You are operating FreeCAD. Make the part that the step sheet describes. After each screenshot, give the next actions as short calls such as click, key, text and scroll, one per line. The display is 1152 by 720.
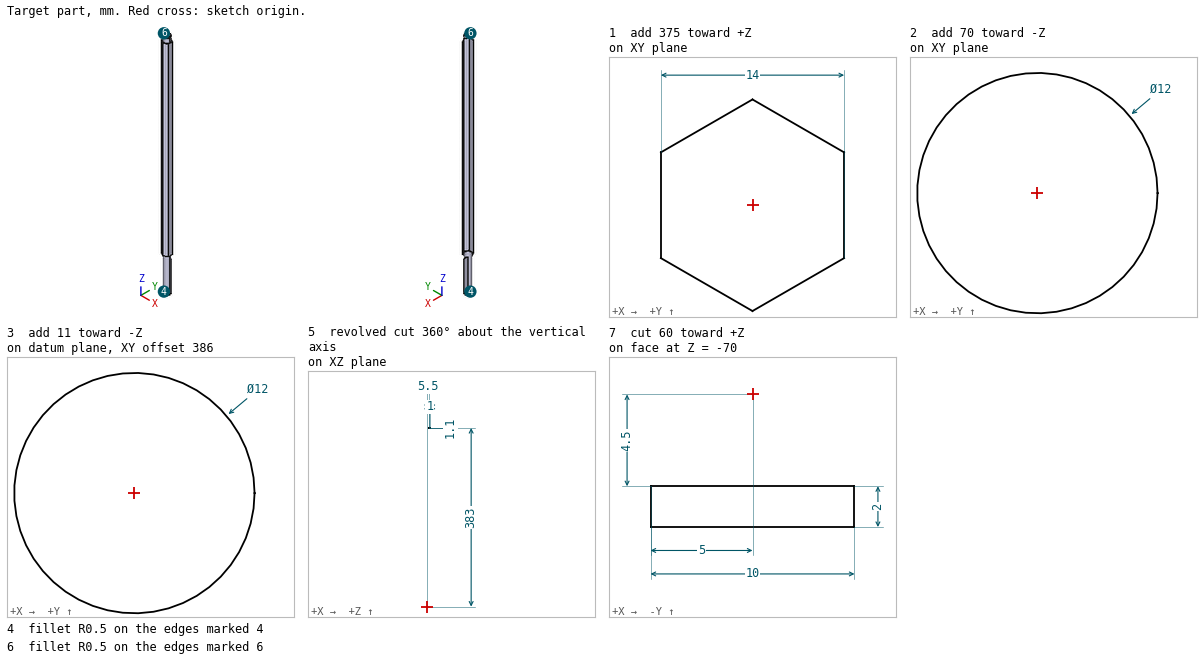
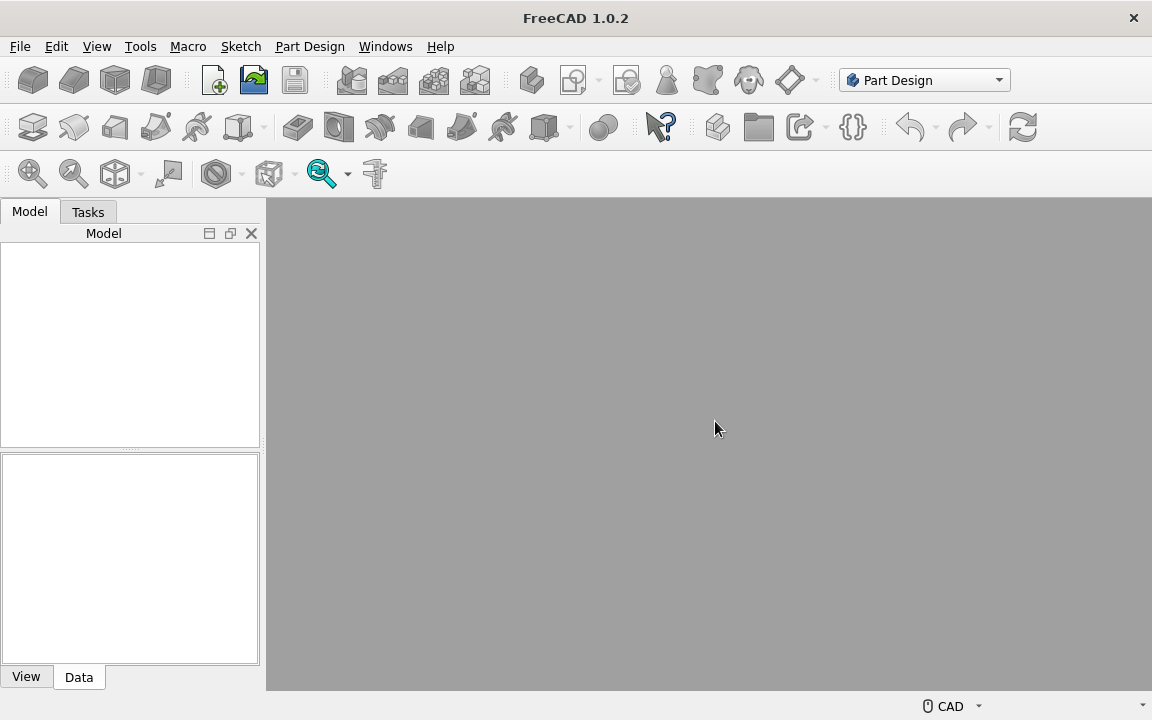
click(213, 80)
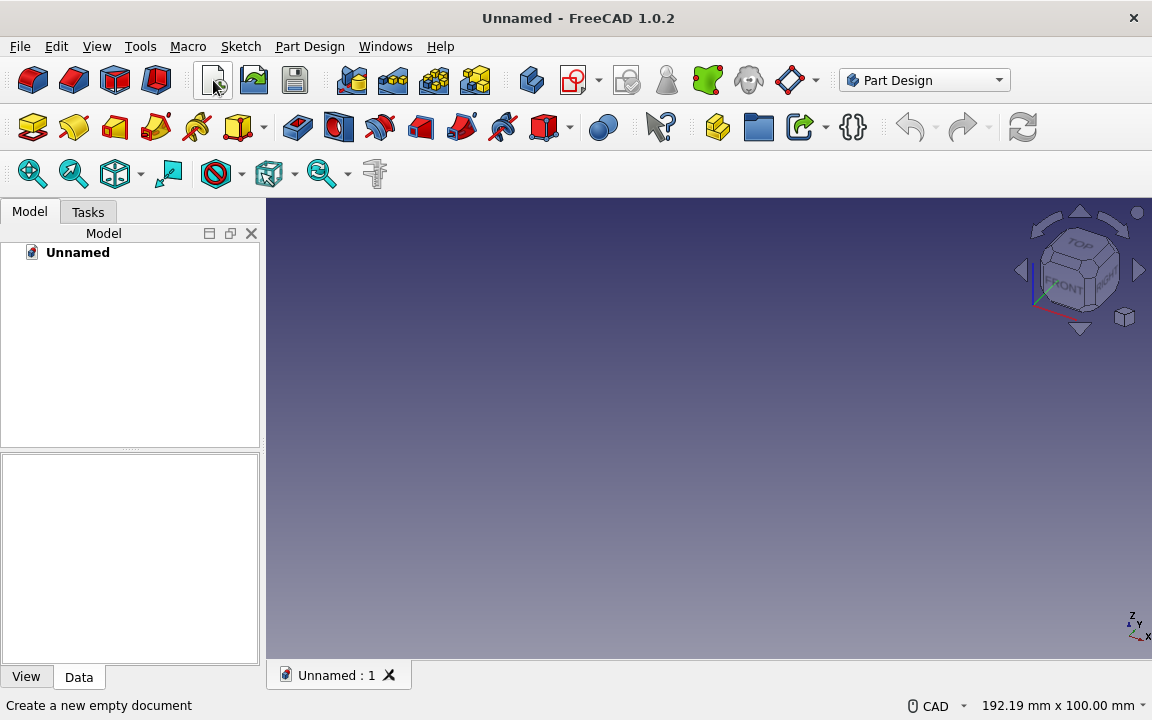
click(572, 80)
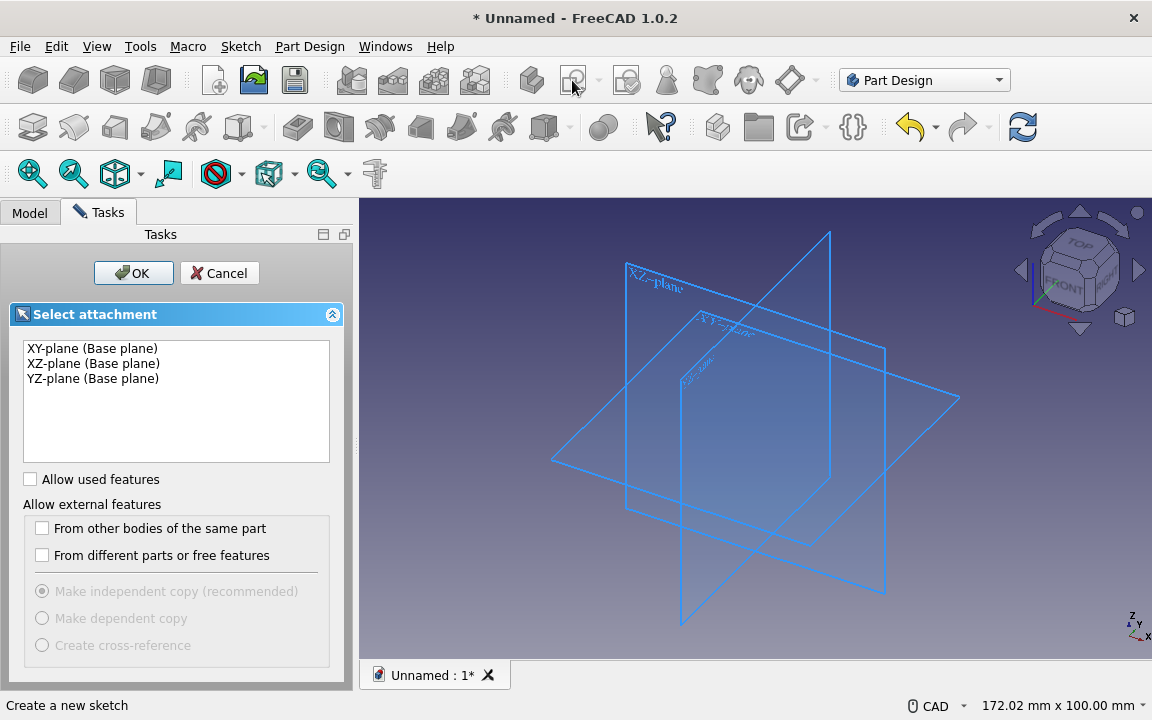
click(84, 348)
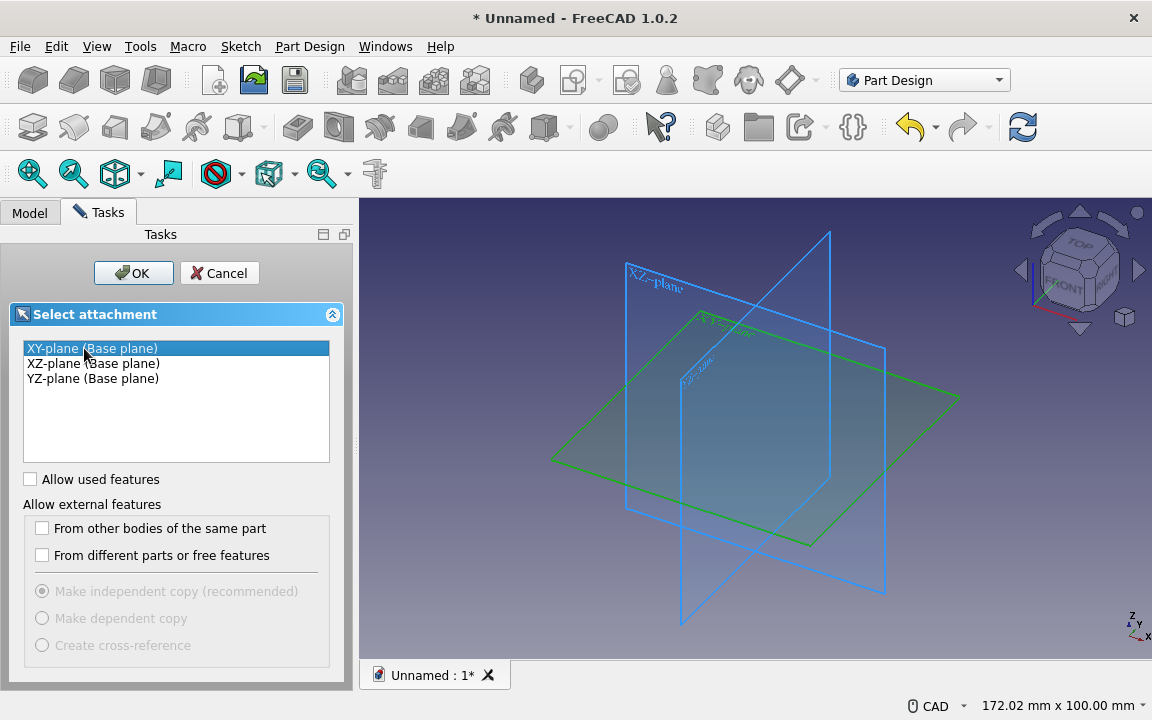
click(134, 273)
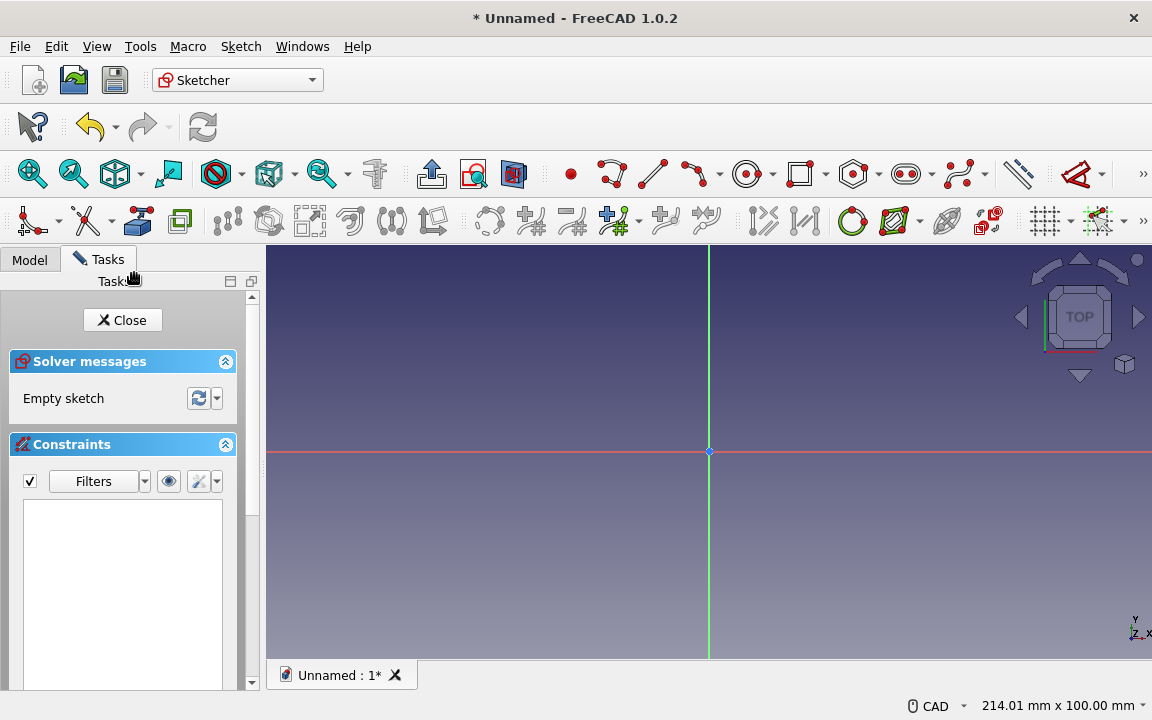
scroll(731, 452, up, 7)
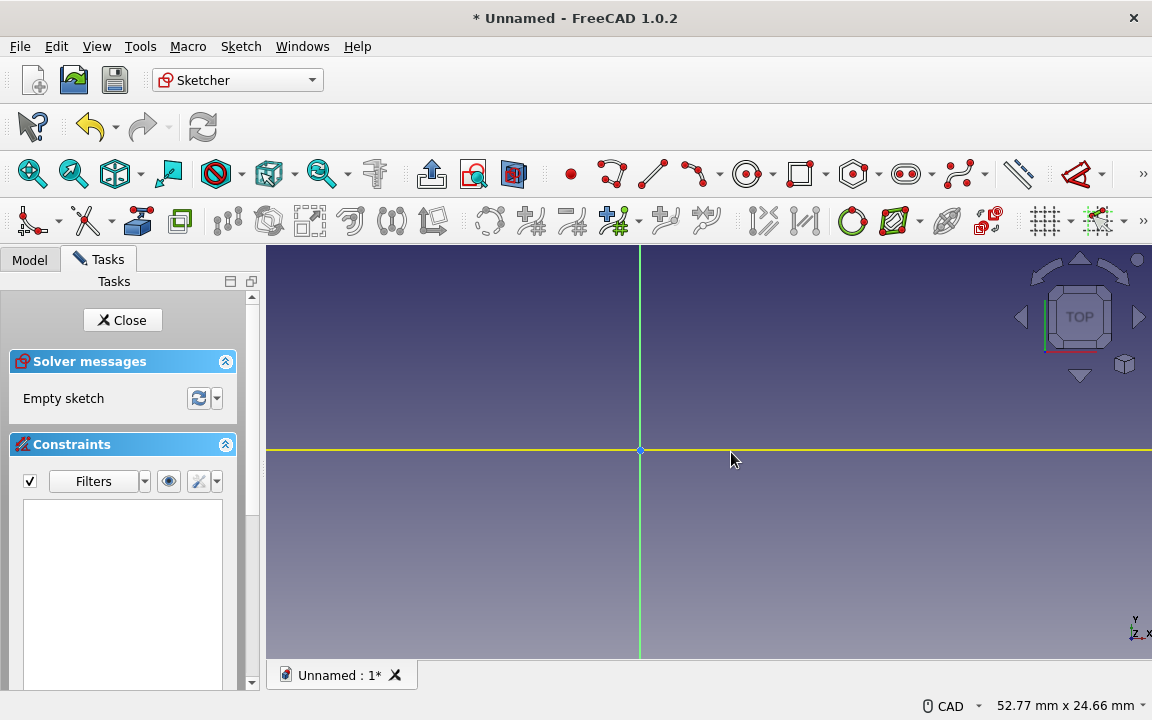
click(852, 174)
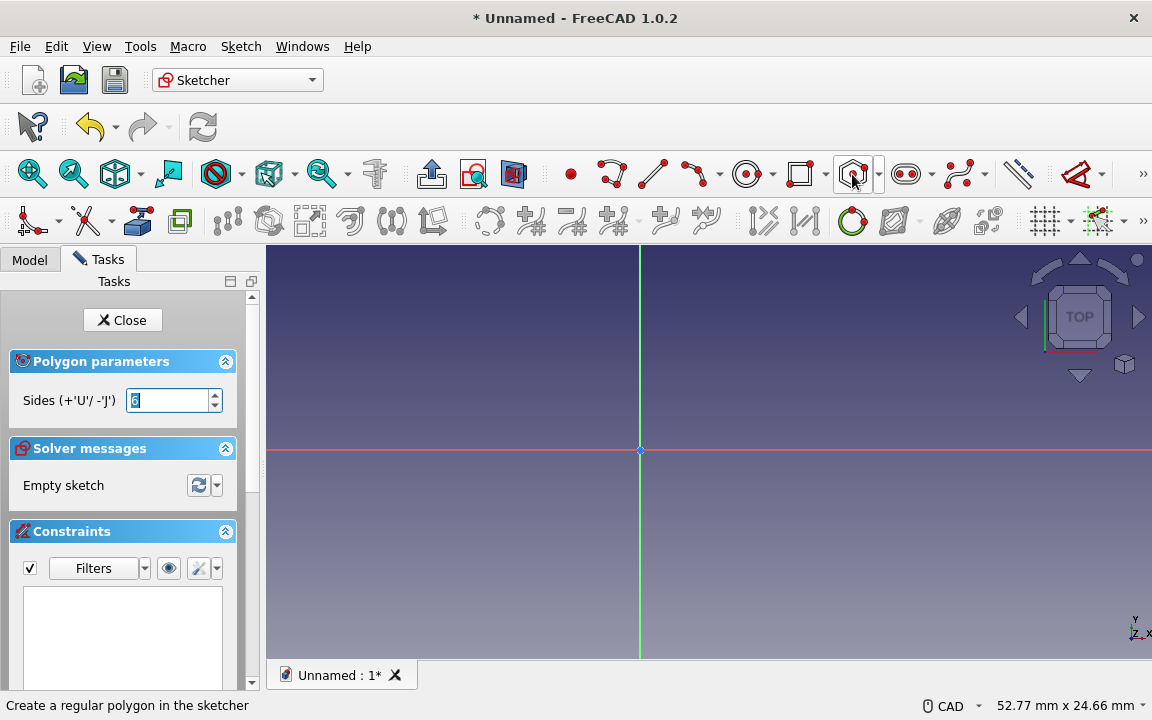
click(640, 450)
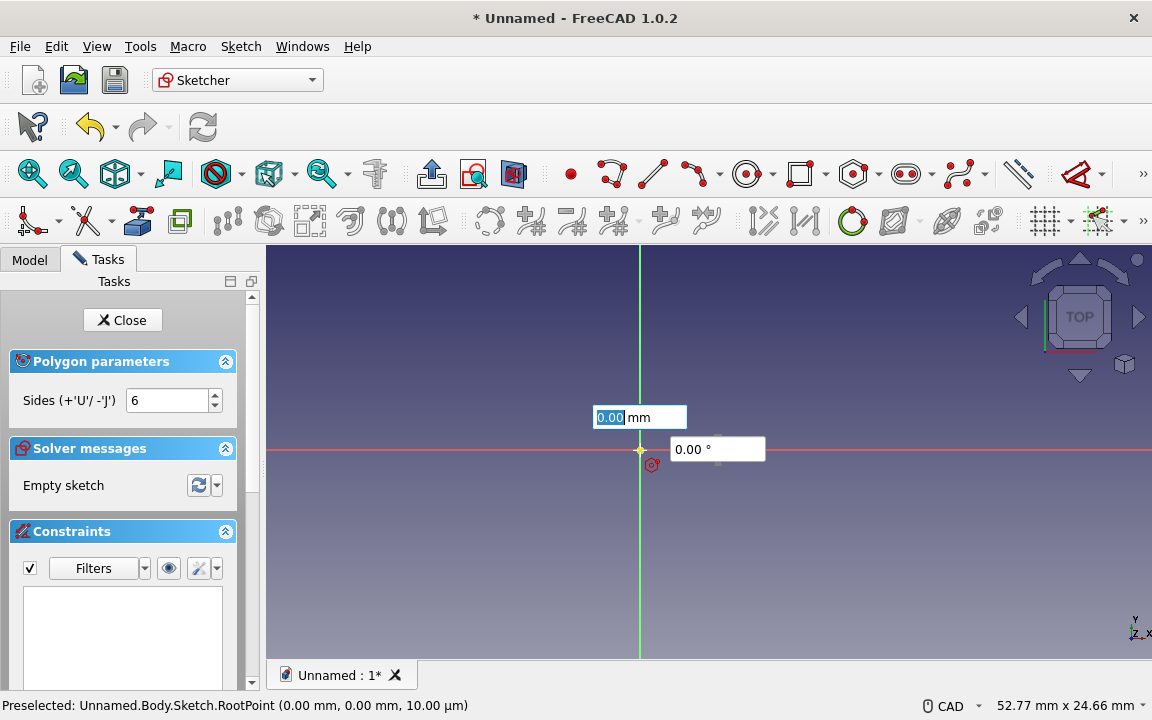
click(640, 315)
key(Escape)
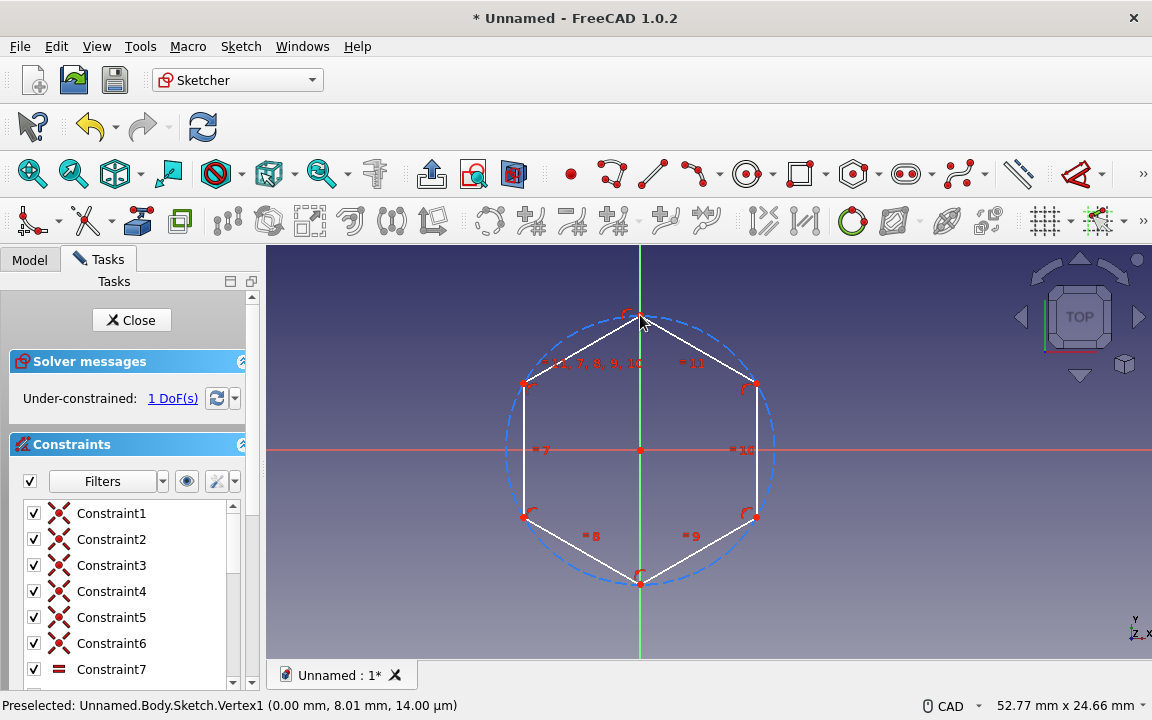
click(1076, 174)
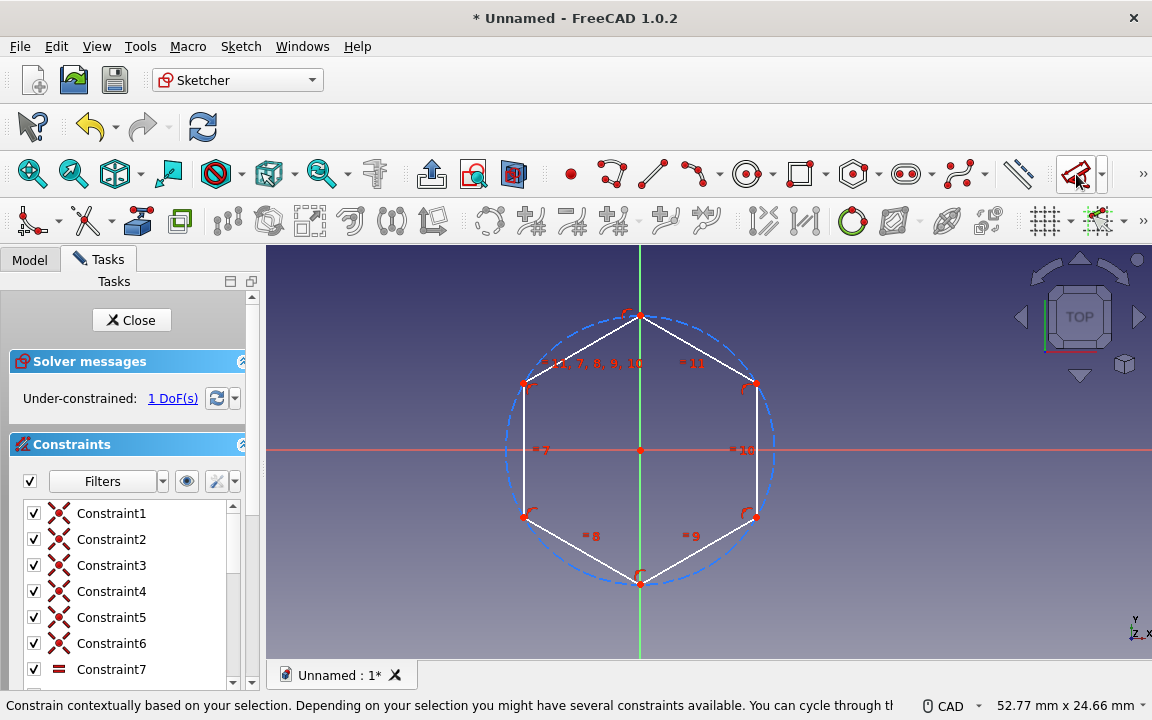
click(524, 383)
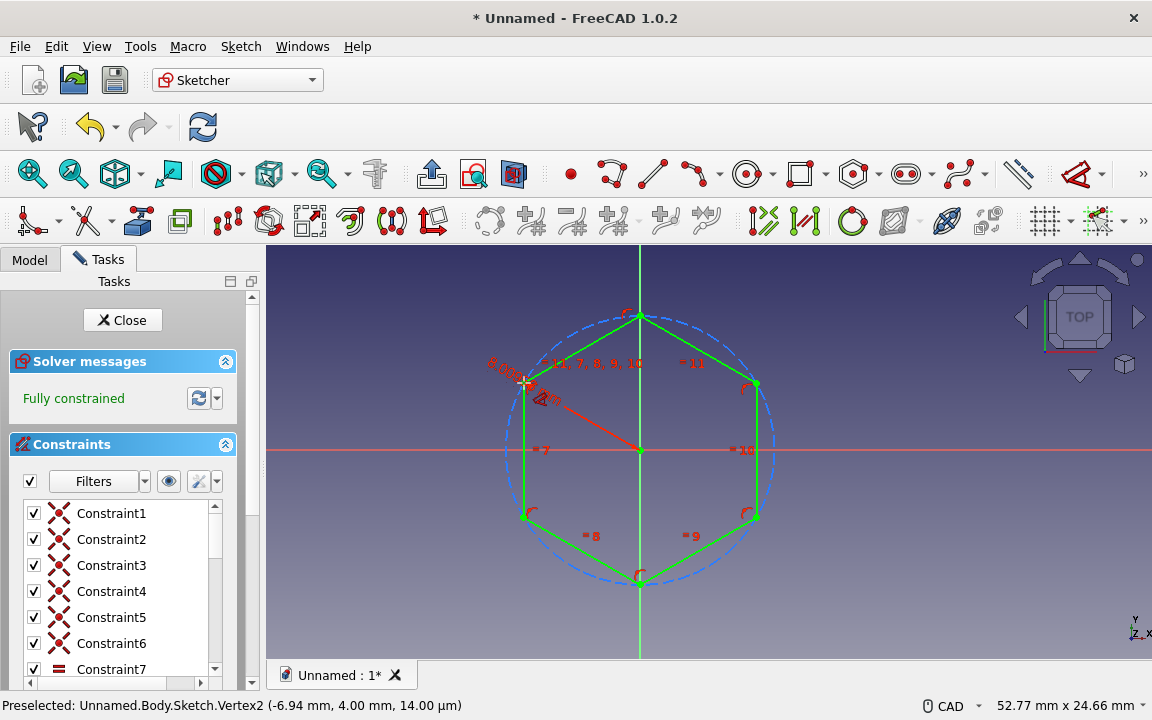
click(757, 518)
click(559, 576)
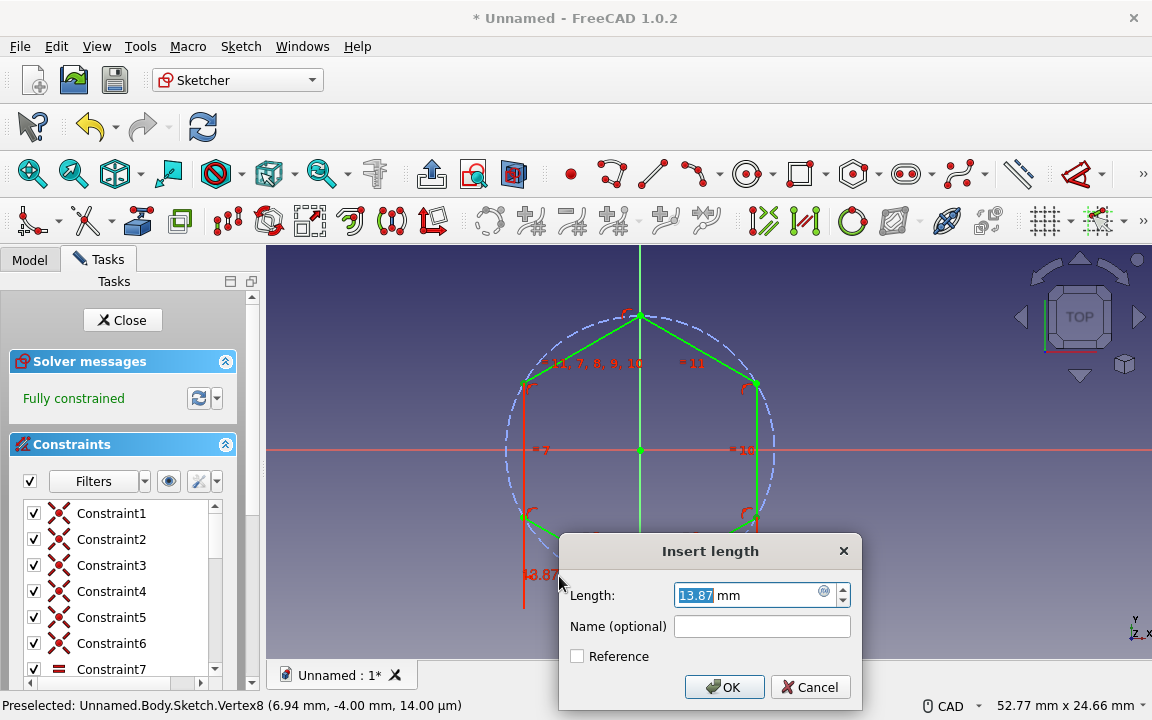
text(14)
key(Return)
key(Escape)